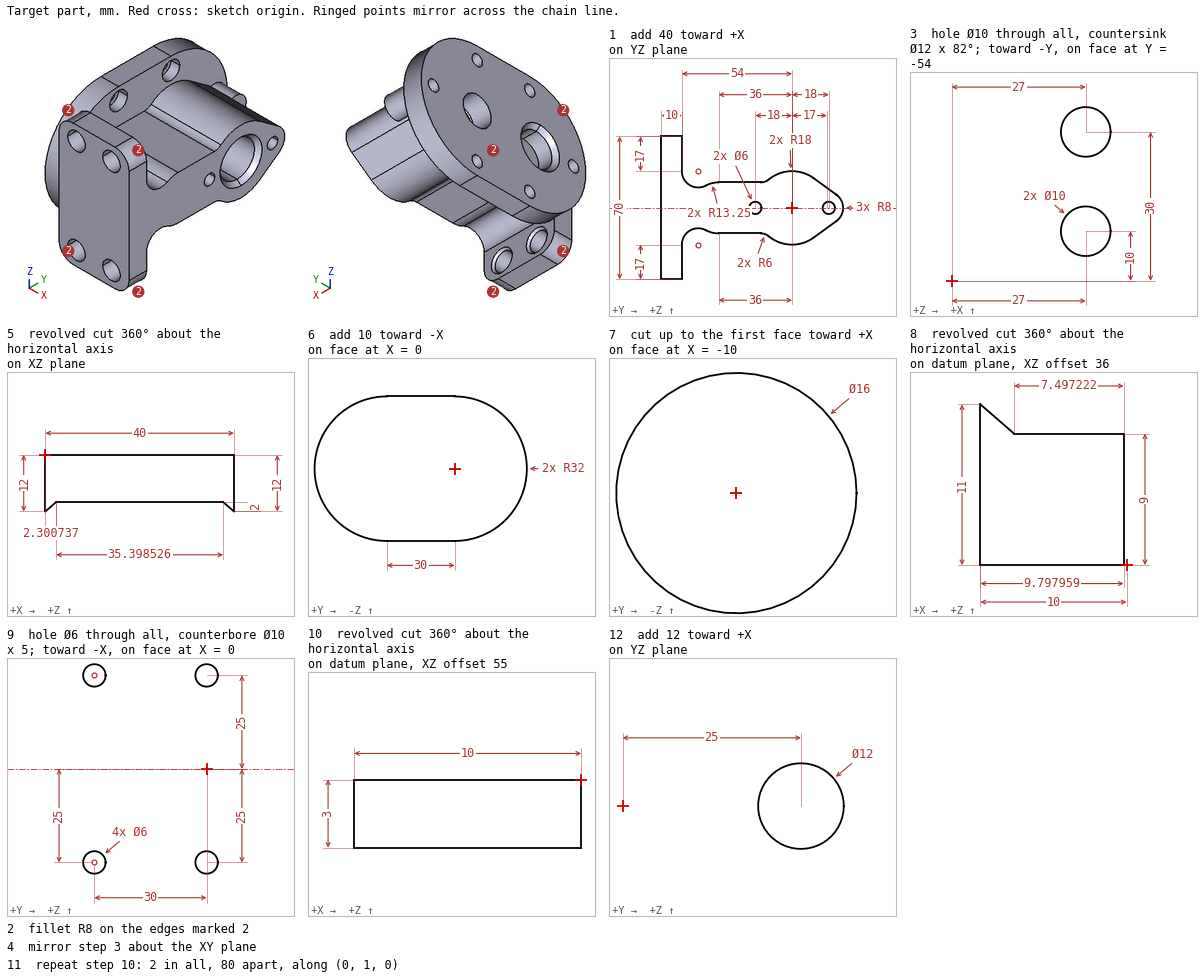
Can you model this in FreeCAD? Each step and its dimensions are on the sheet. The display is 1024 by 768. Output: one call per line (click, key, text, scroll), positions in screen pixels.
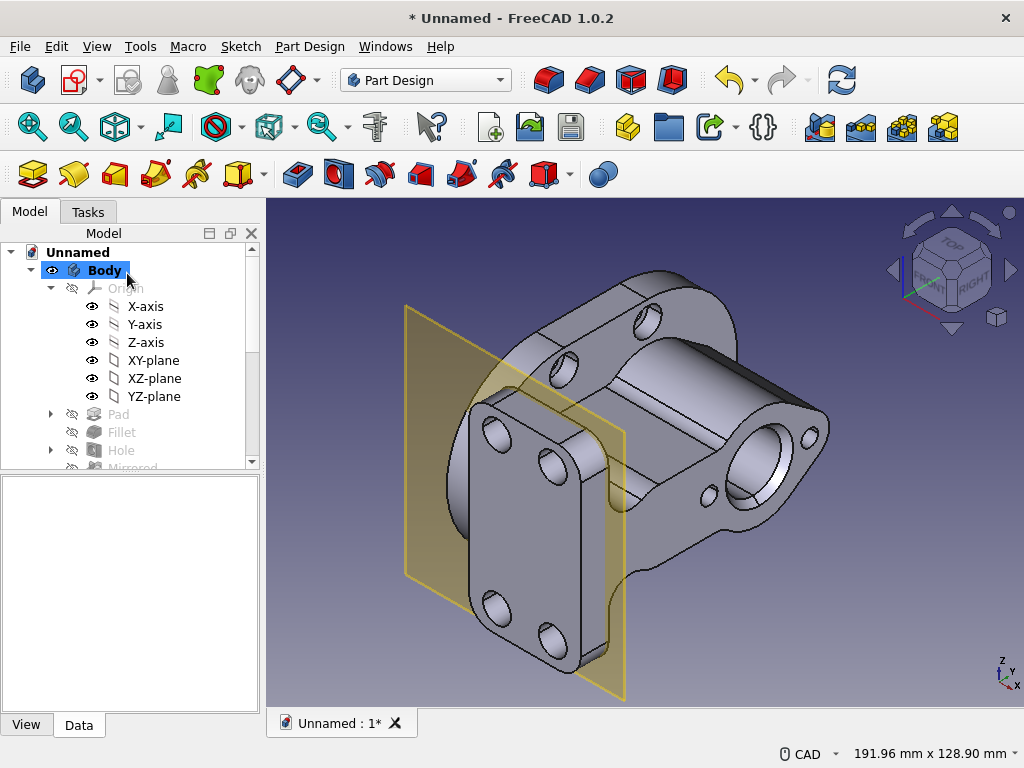
scroll(101, 356, down, 3)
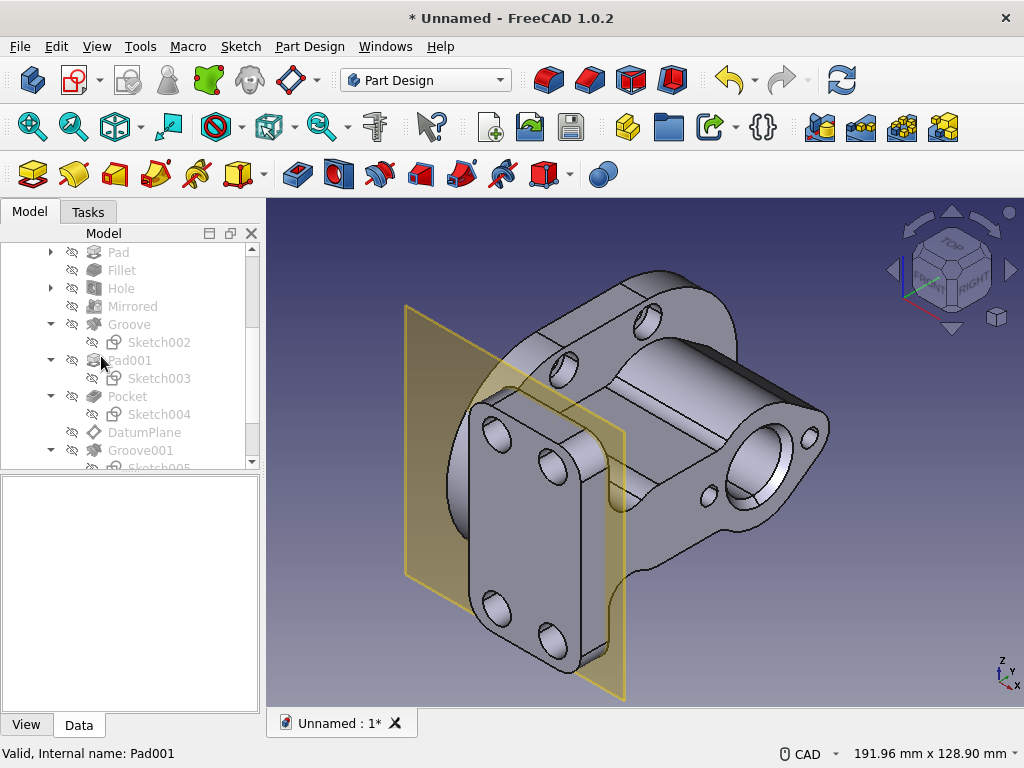
scroll(141, 356, up, 15)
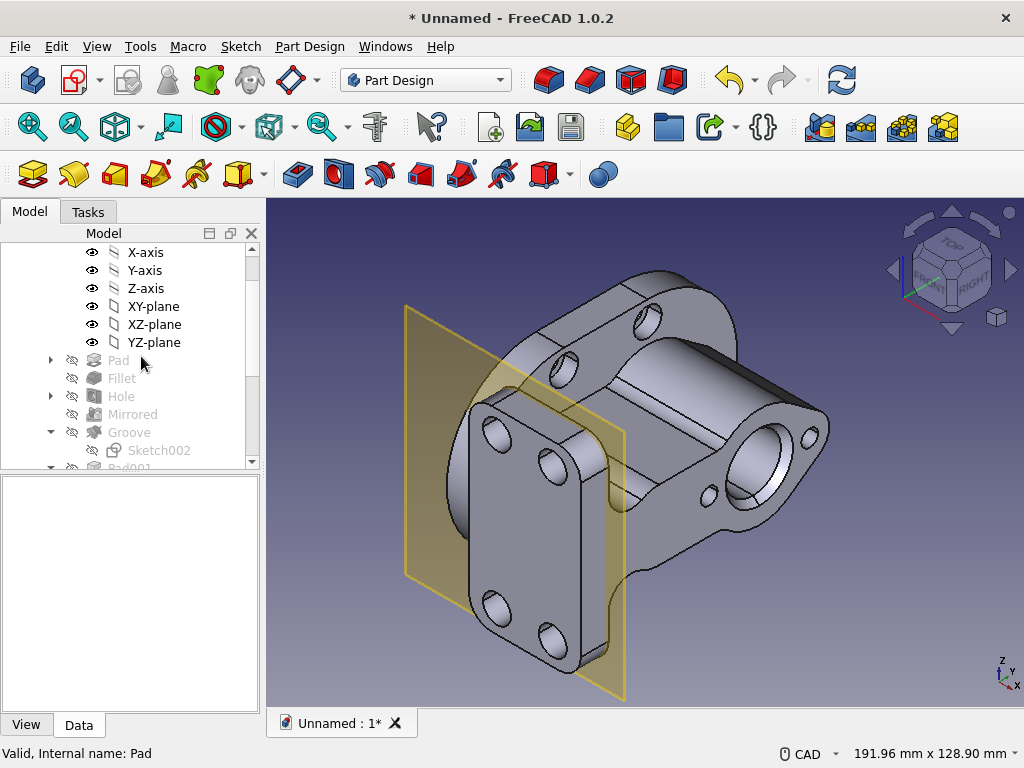
scroll(101, 356, down, 6)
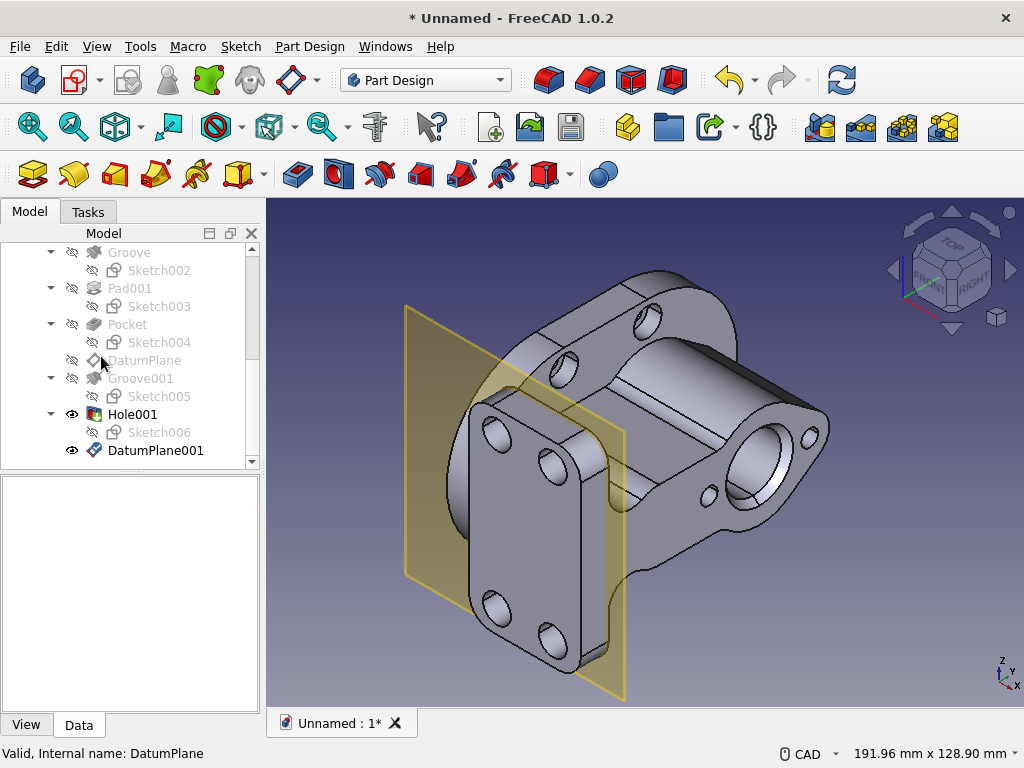
click(117, 450)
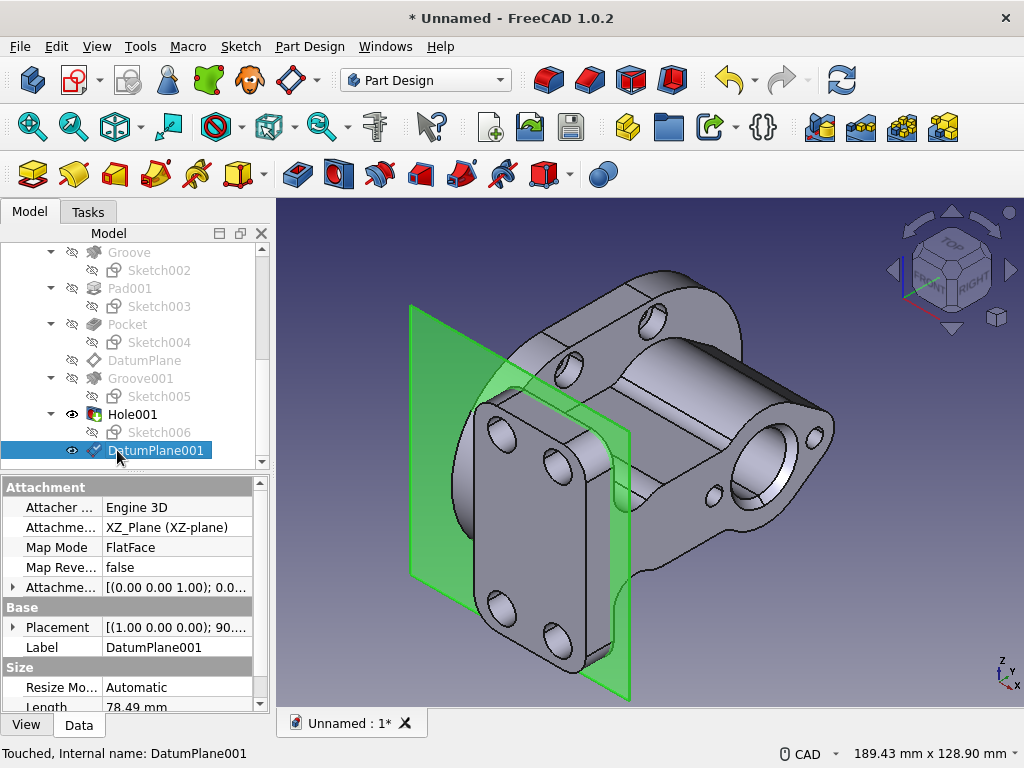
click(74, 80)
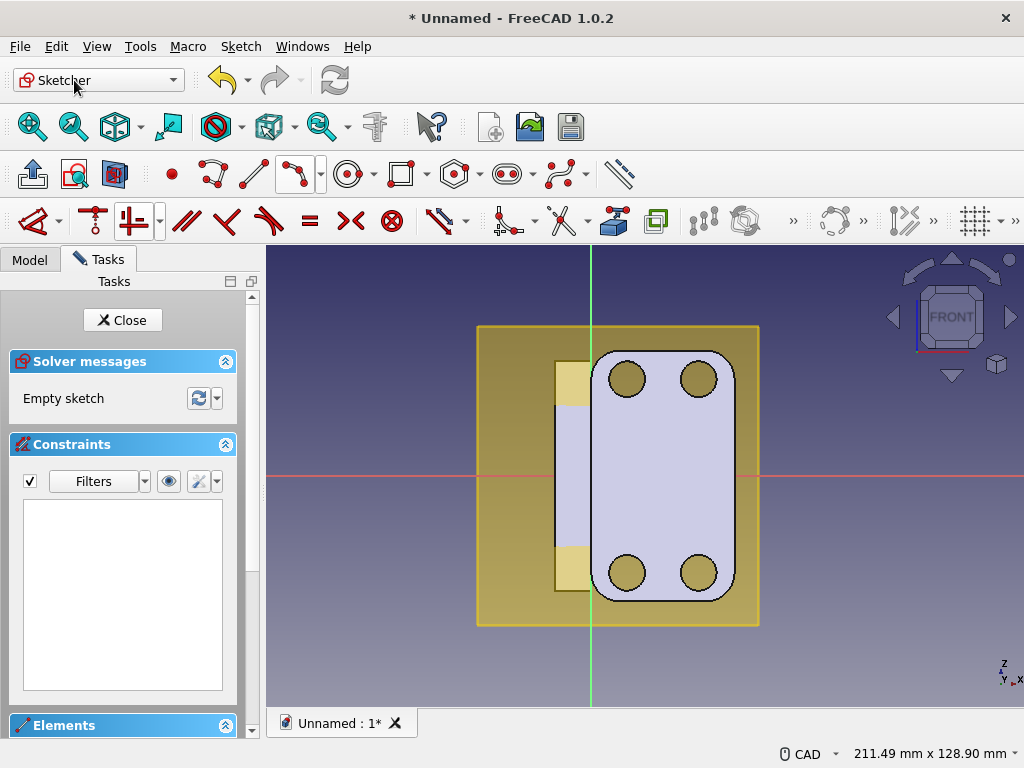
click(115, 174)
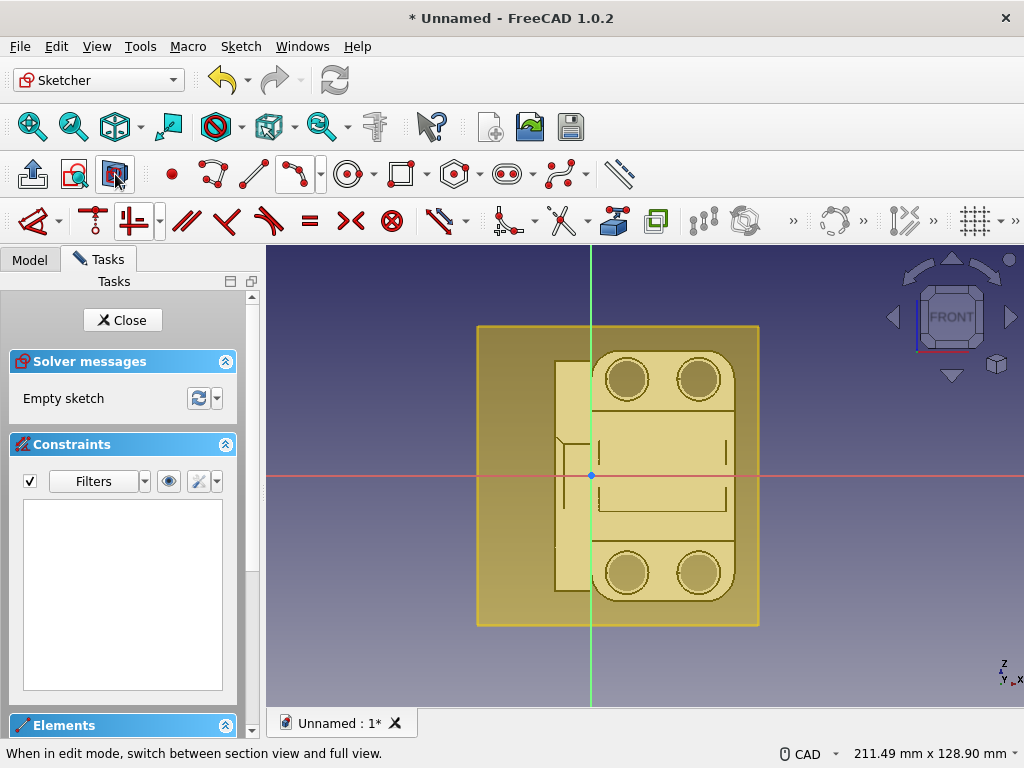
scroll(573, 482, up, 12)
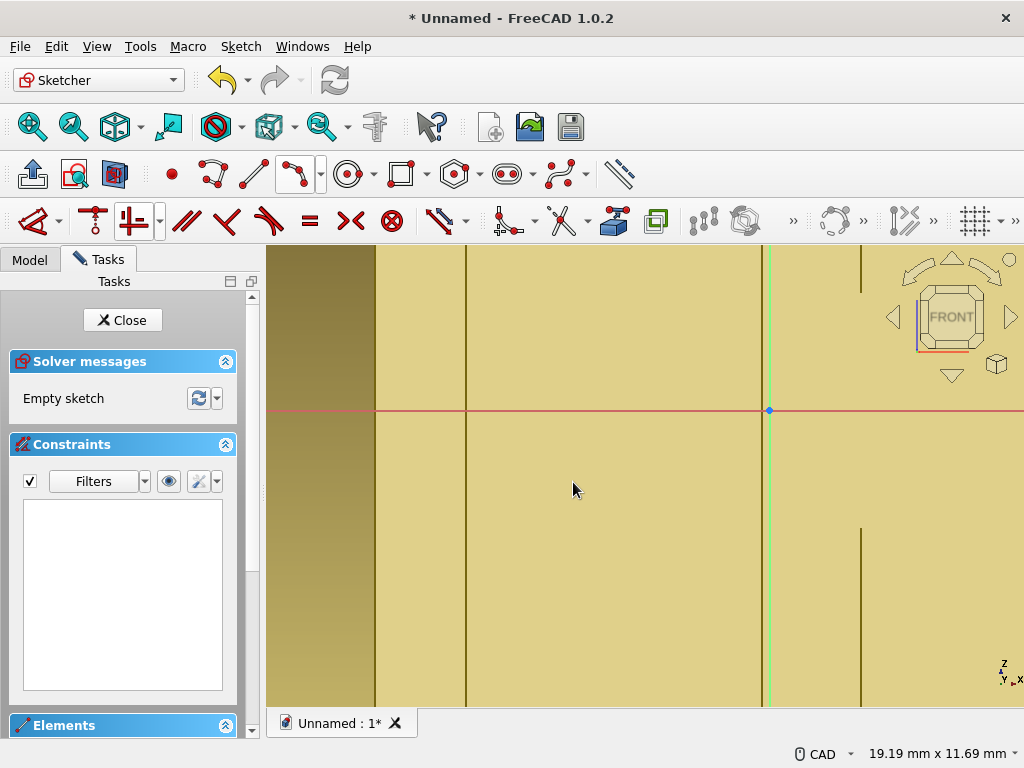
click(400, 174)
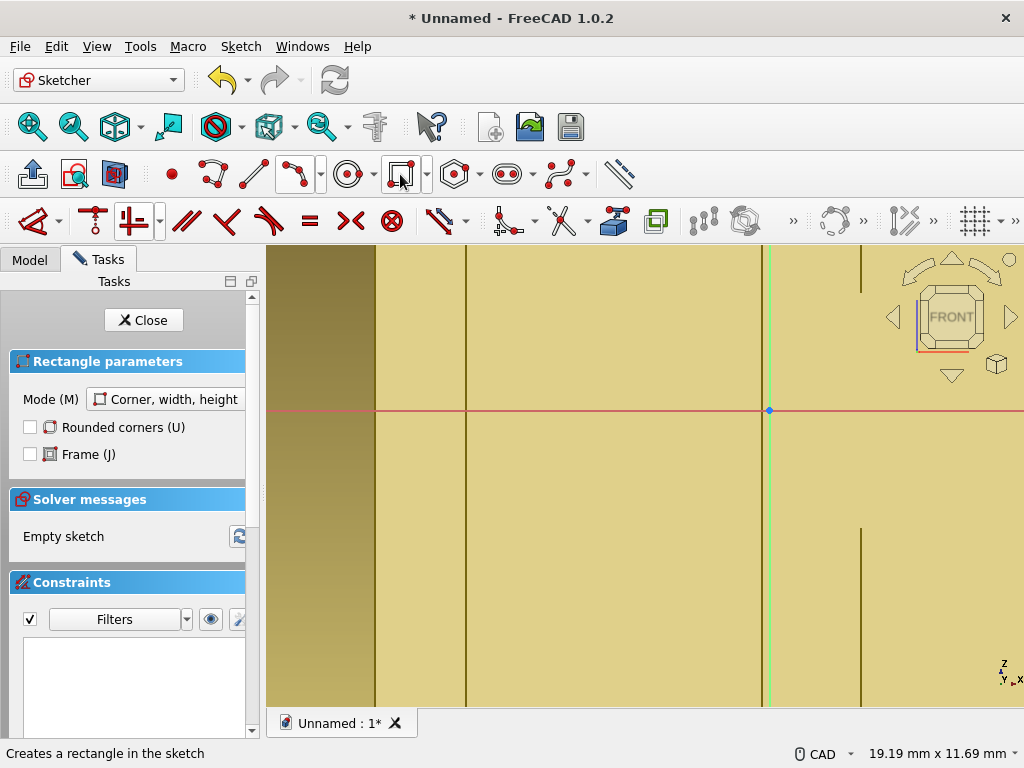
click(770, 411)
click(375, 529)
key(Escape)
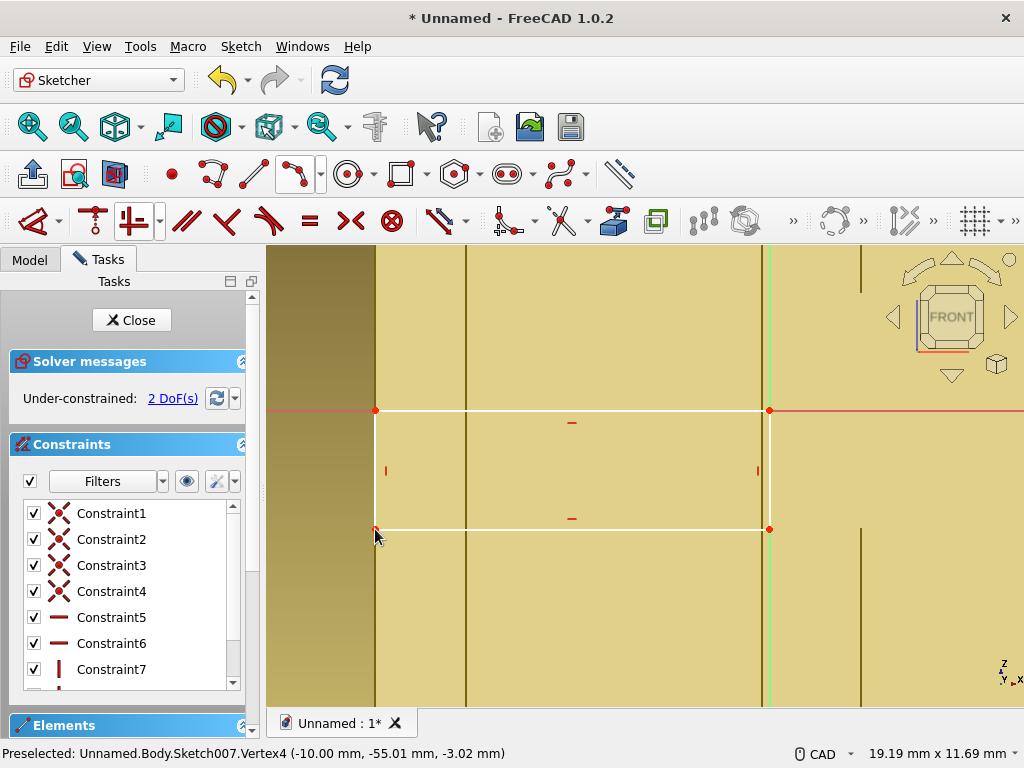
click(32, 222)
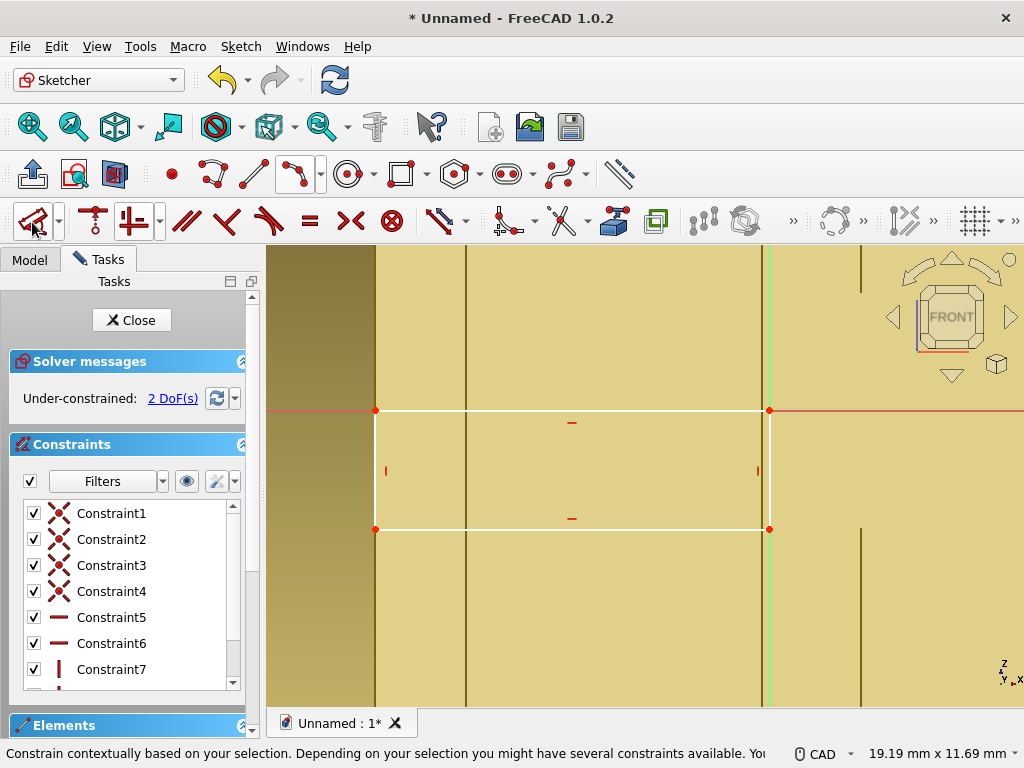
click(375, 446)
click(341, 470)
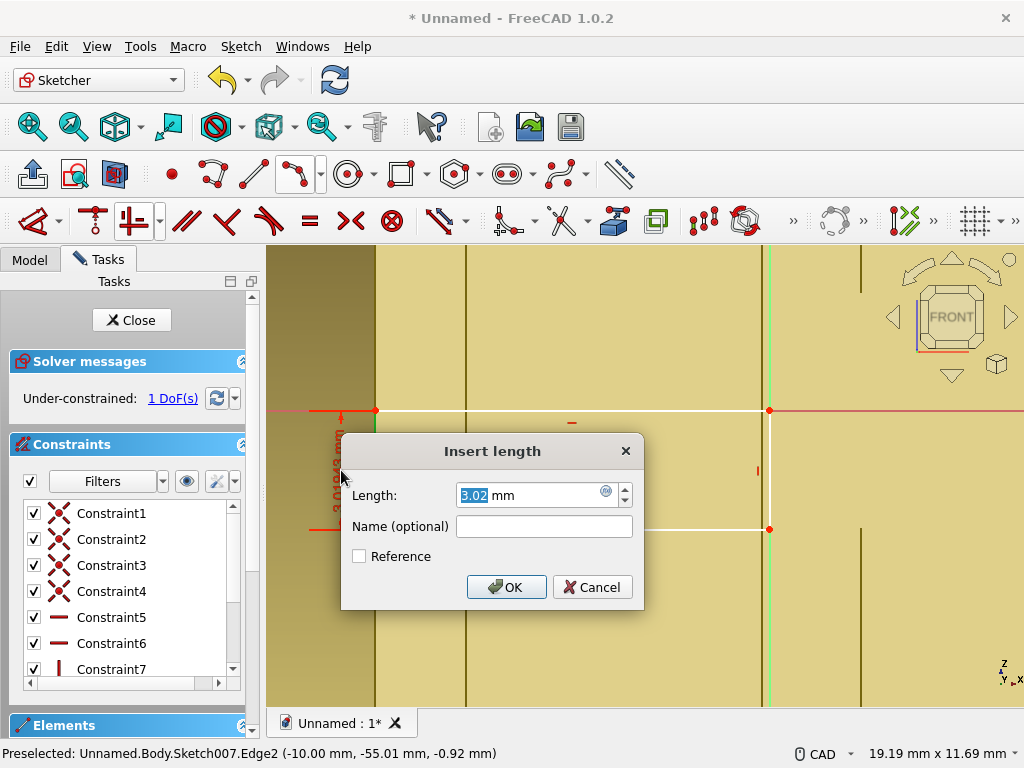
text(3)
key(Return)